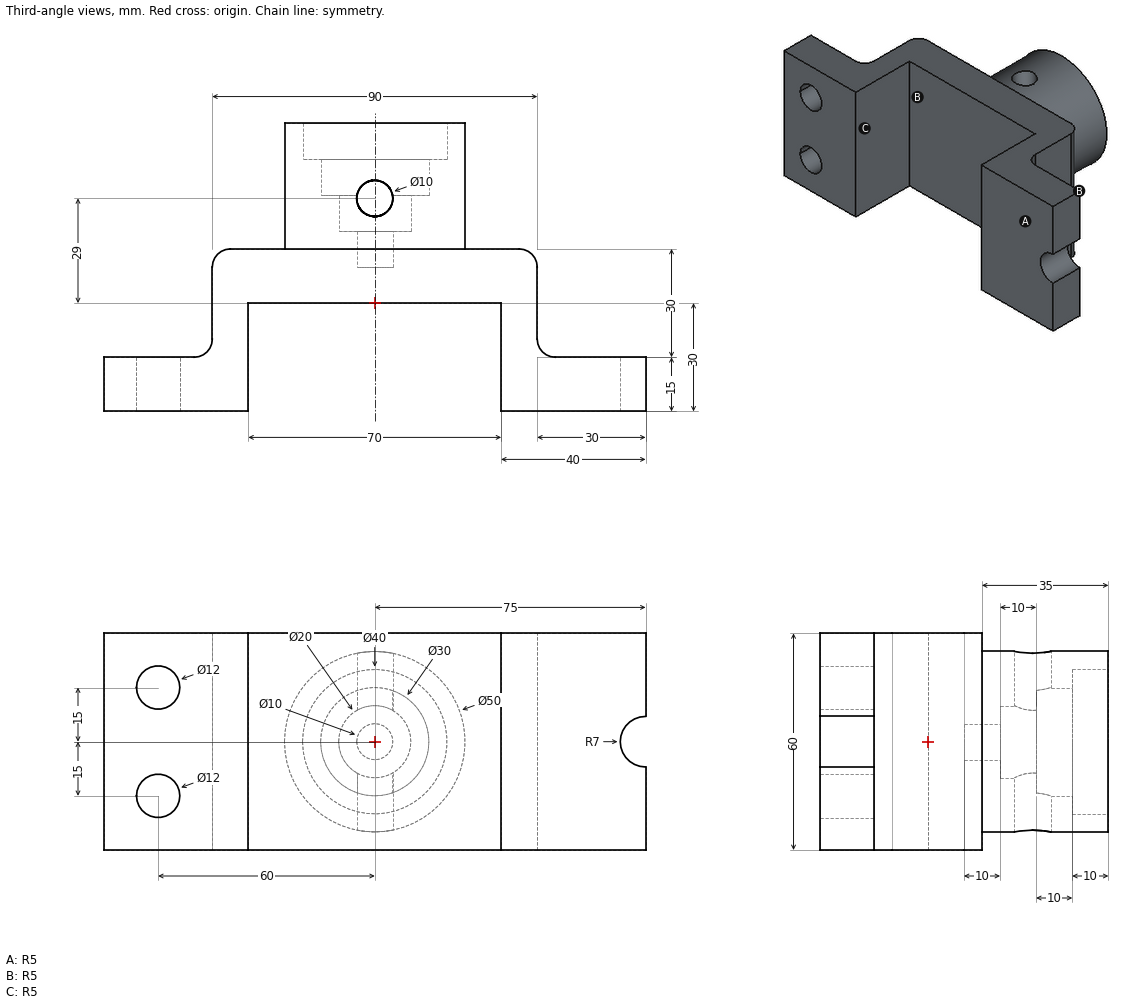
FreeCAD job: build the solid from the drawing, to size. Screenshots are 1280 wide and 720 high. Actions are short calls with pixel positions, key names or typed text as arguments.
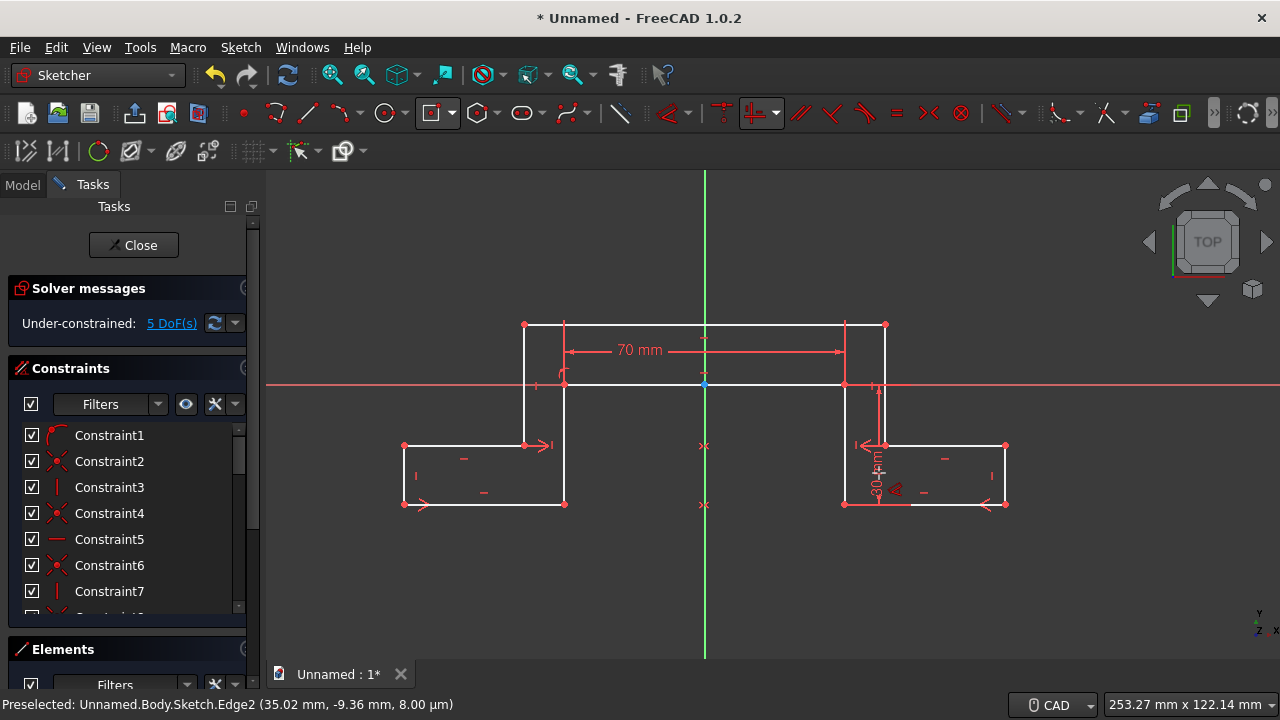
click(893, 505)
click(925, 539)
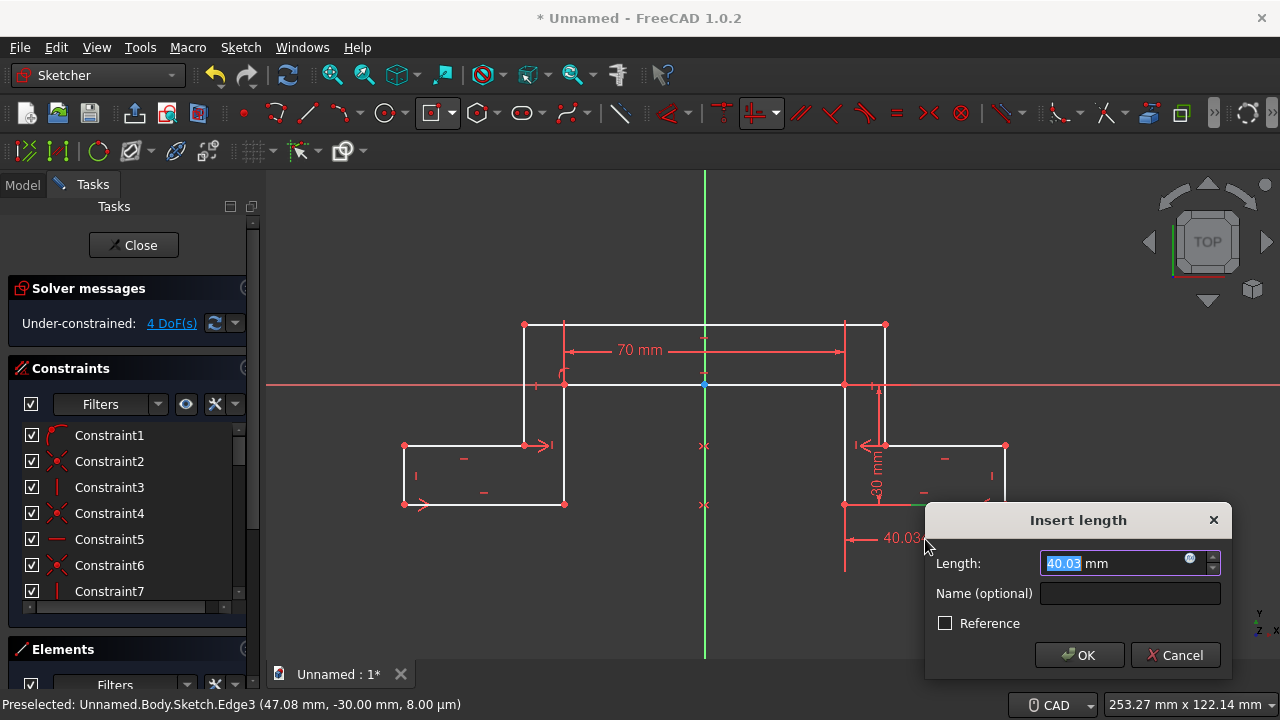
text(40)
key(Return)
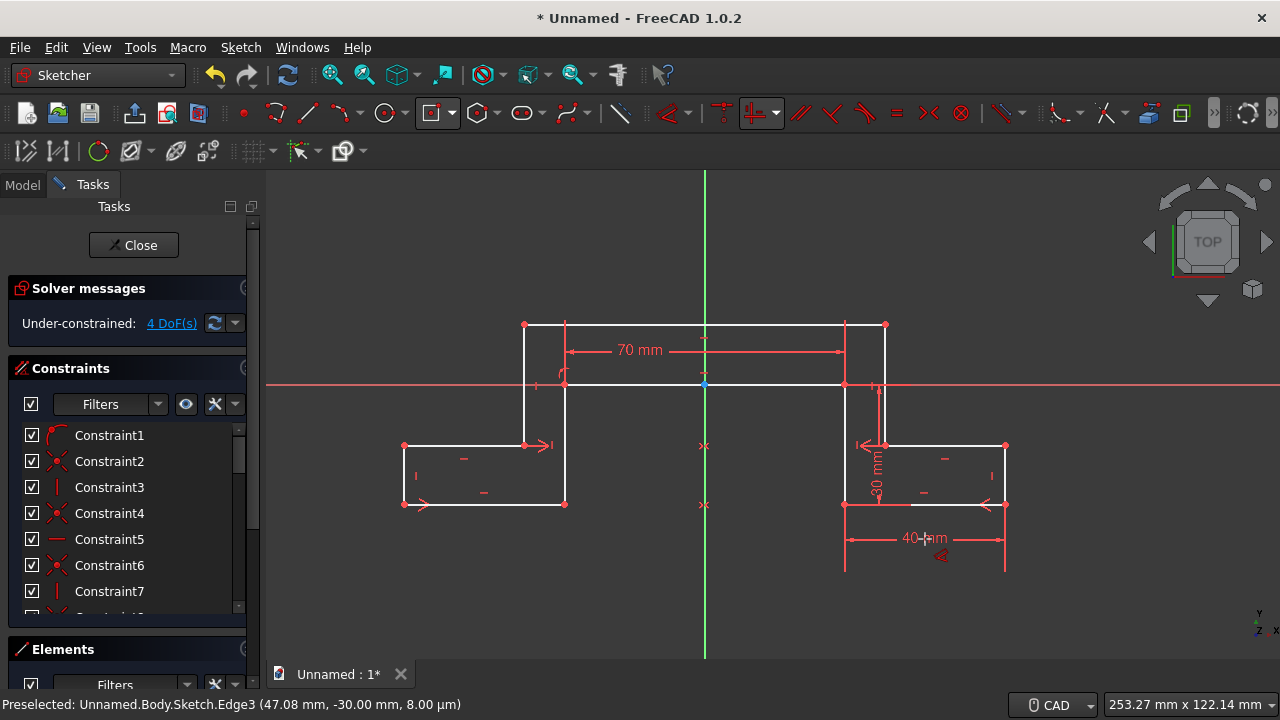
click(1005, 487)
click(1039, 475)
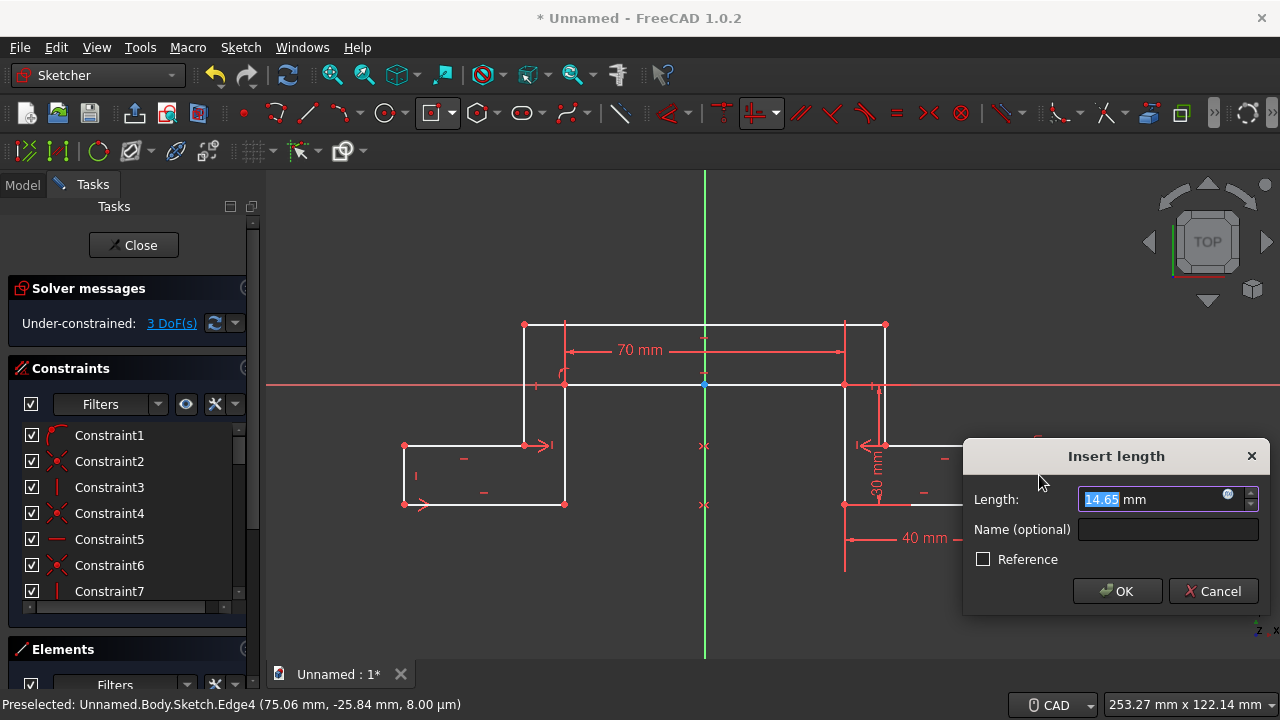
text(15)
key(Return)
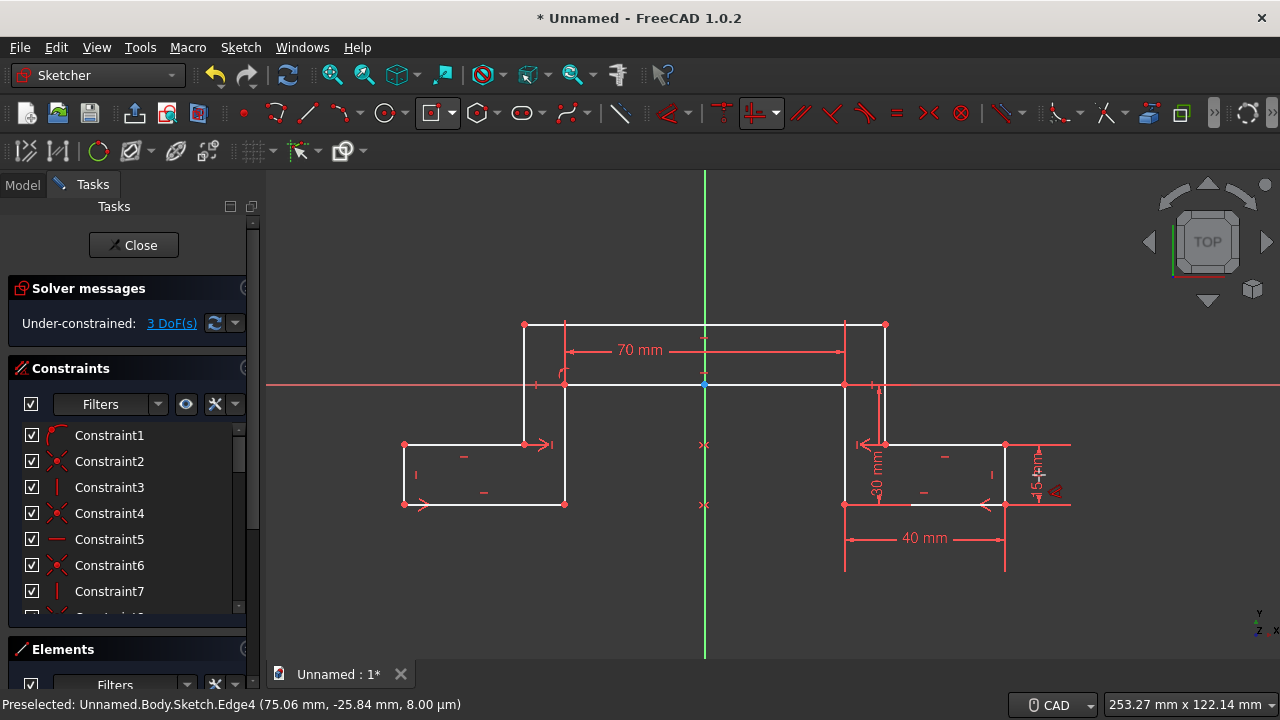
click(969, 445)
click(945, 411)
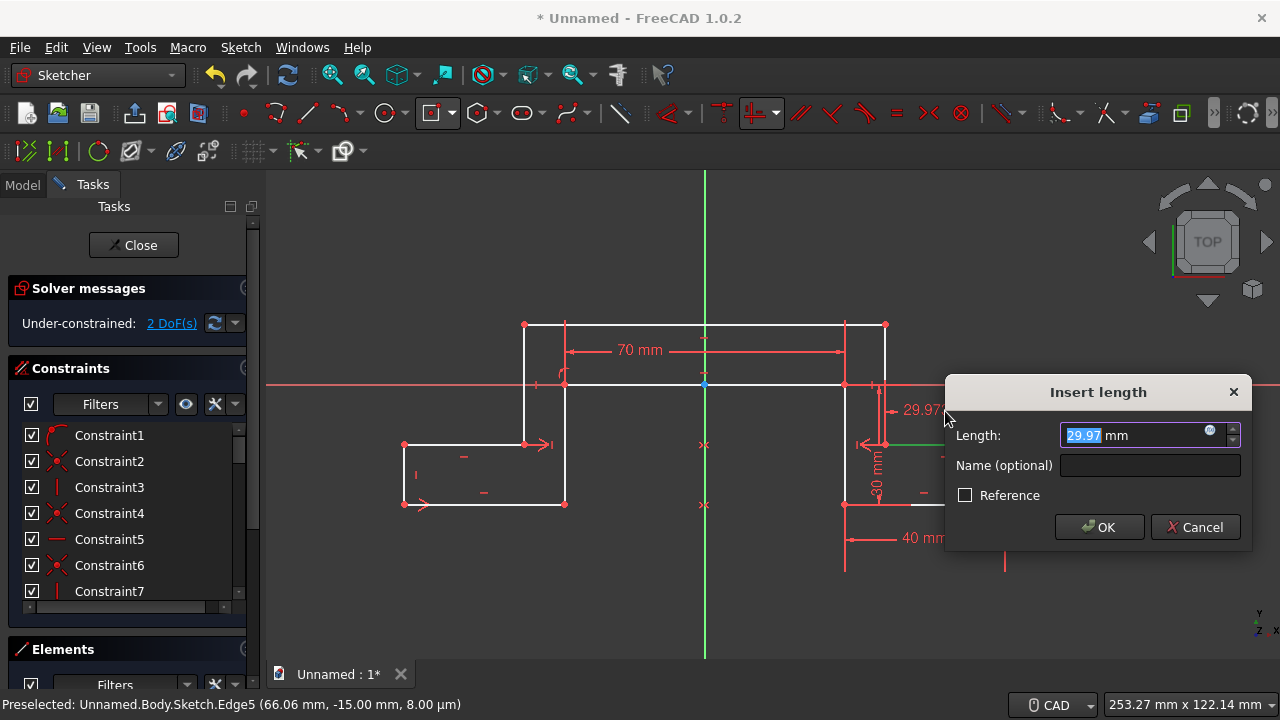
text(30)
key(Return)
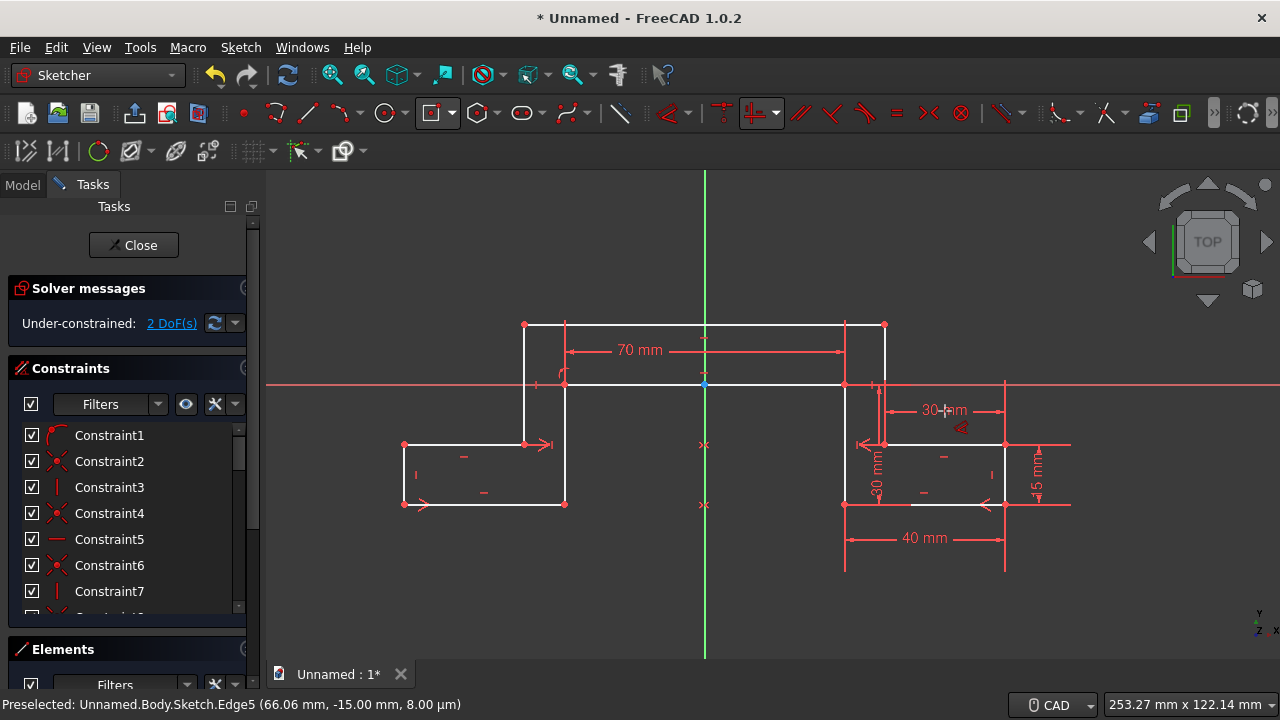
click(885, 409)
click(919, 357)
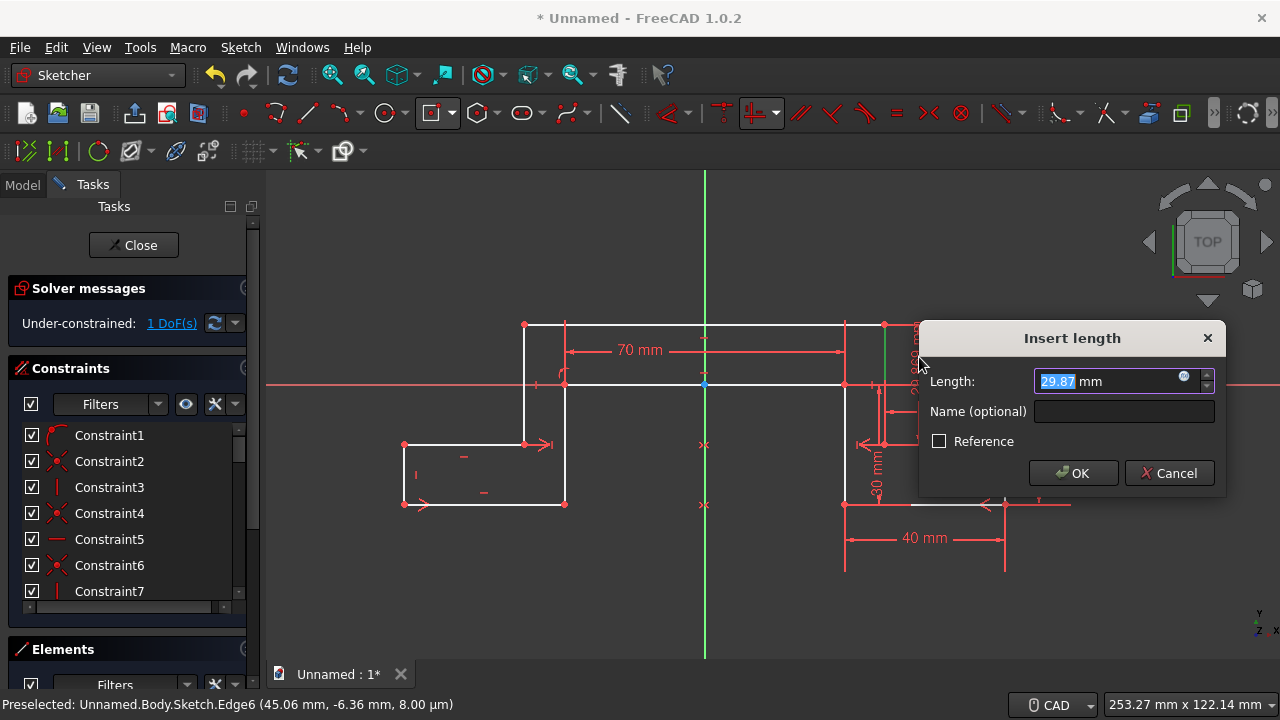
text(30)
key(Return)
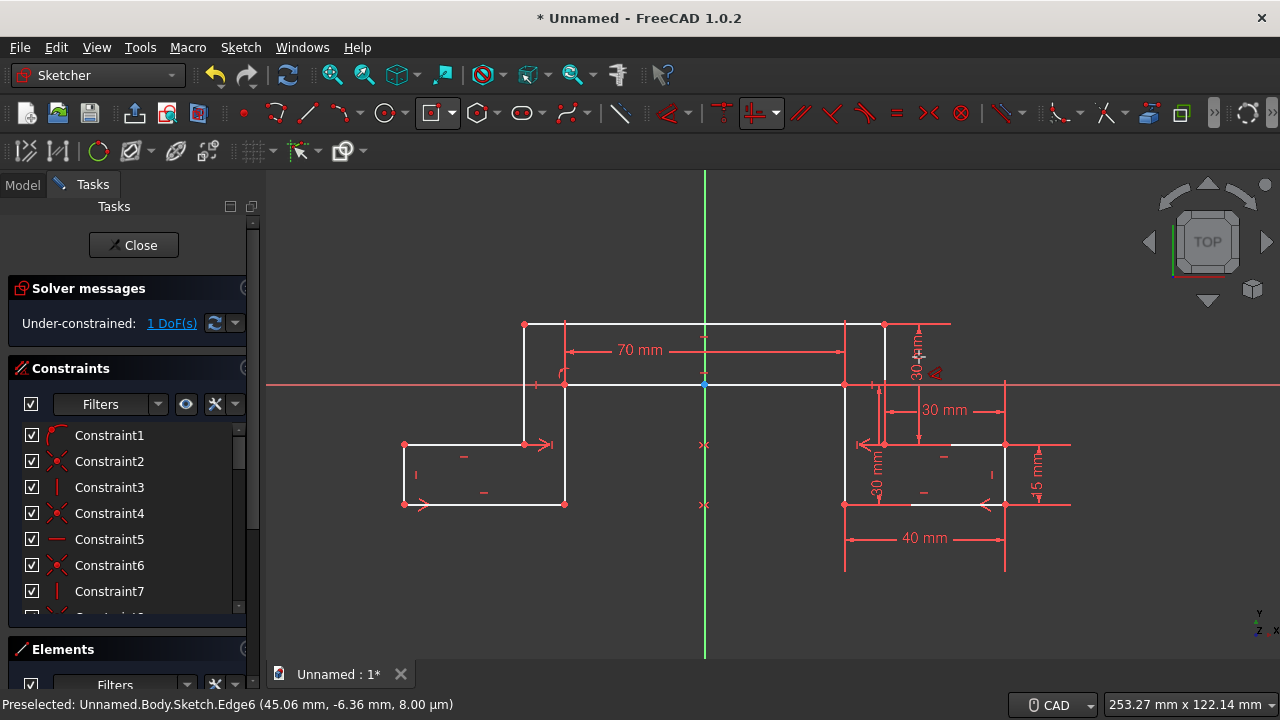
click(777, 324)
click(622, 290)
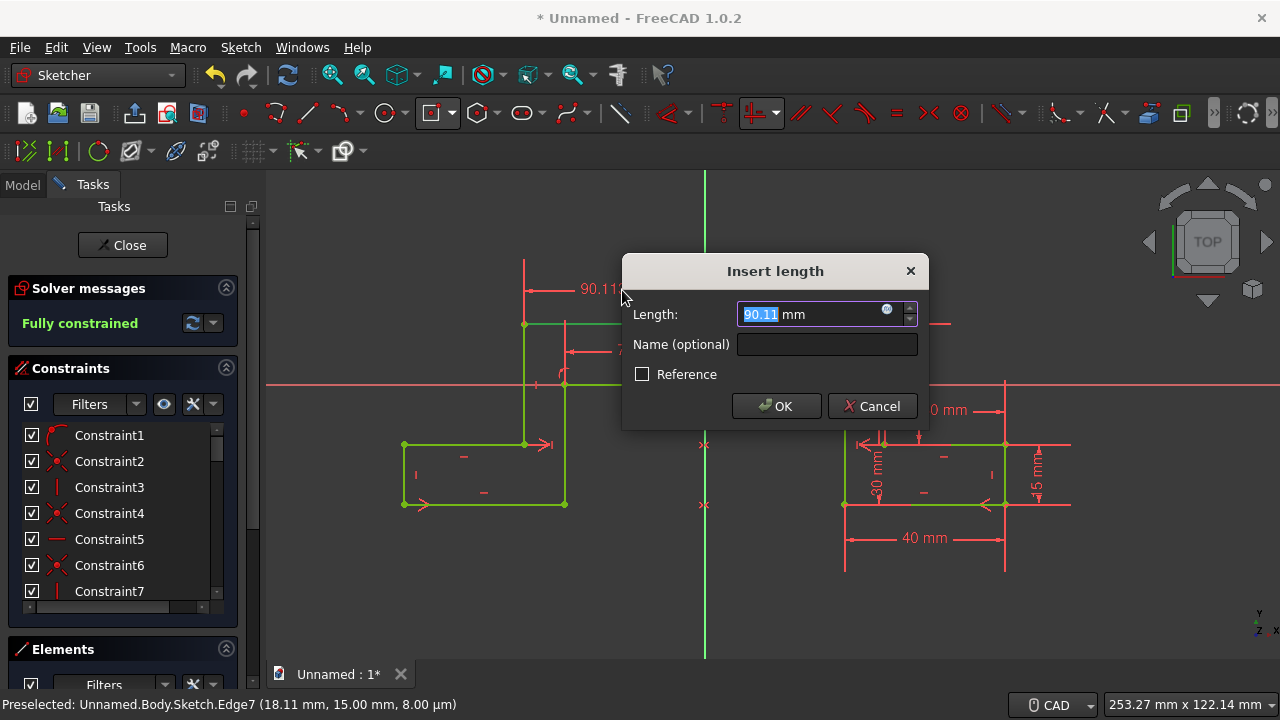
text(90)
key(Return)
key(Escape)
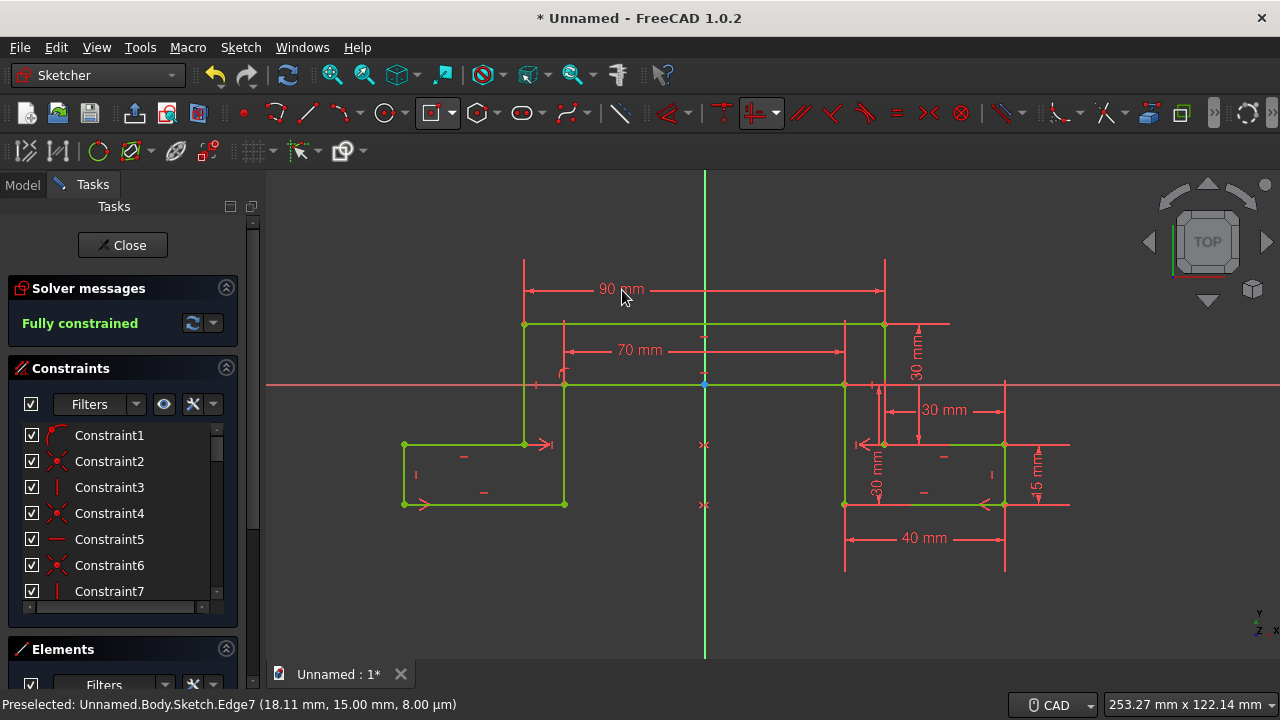
click(123, 245)